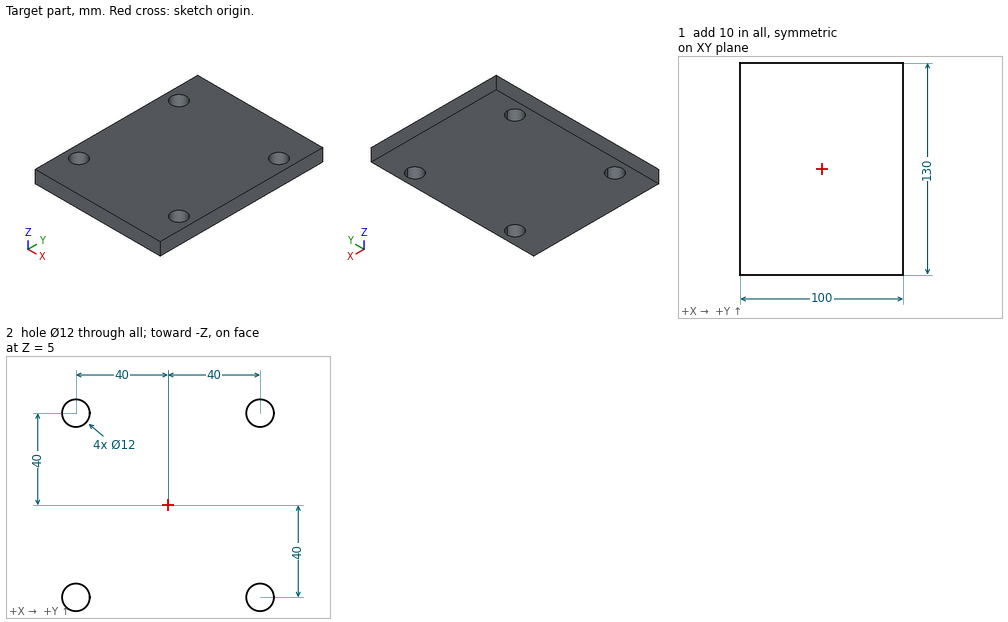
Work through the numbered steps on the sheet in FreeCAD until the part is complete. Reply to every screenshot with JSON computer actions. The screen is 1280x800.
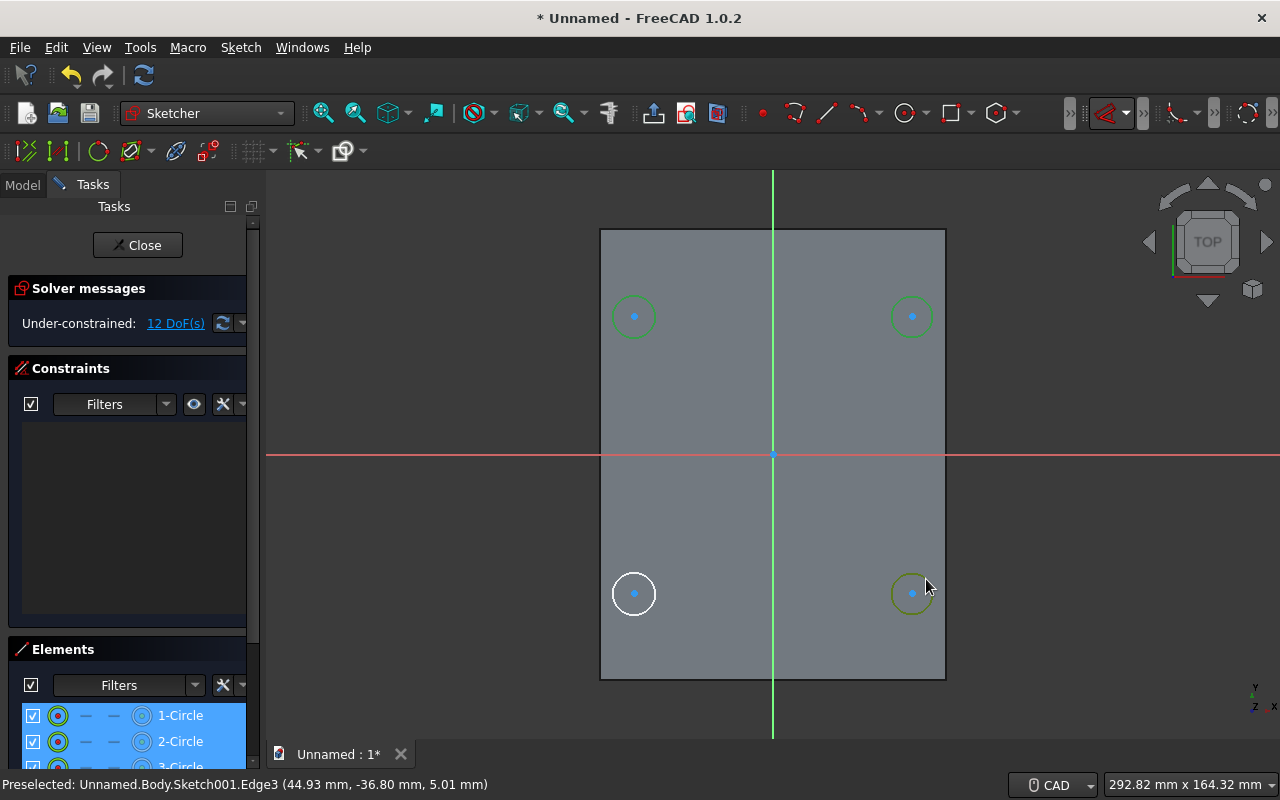
{"action": "left_click", "coordinate": [649, 579]}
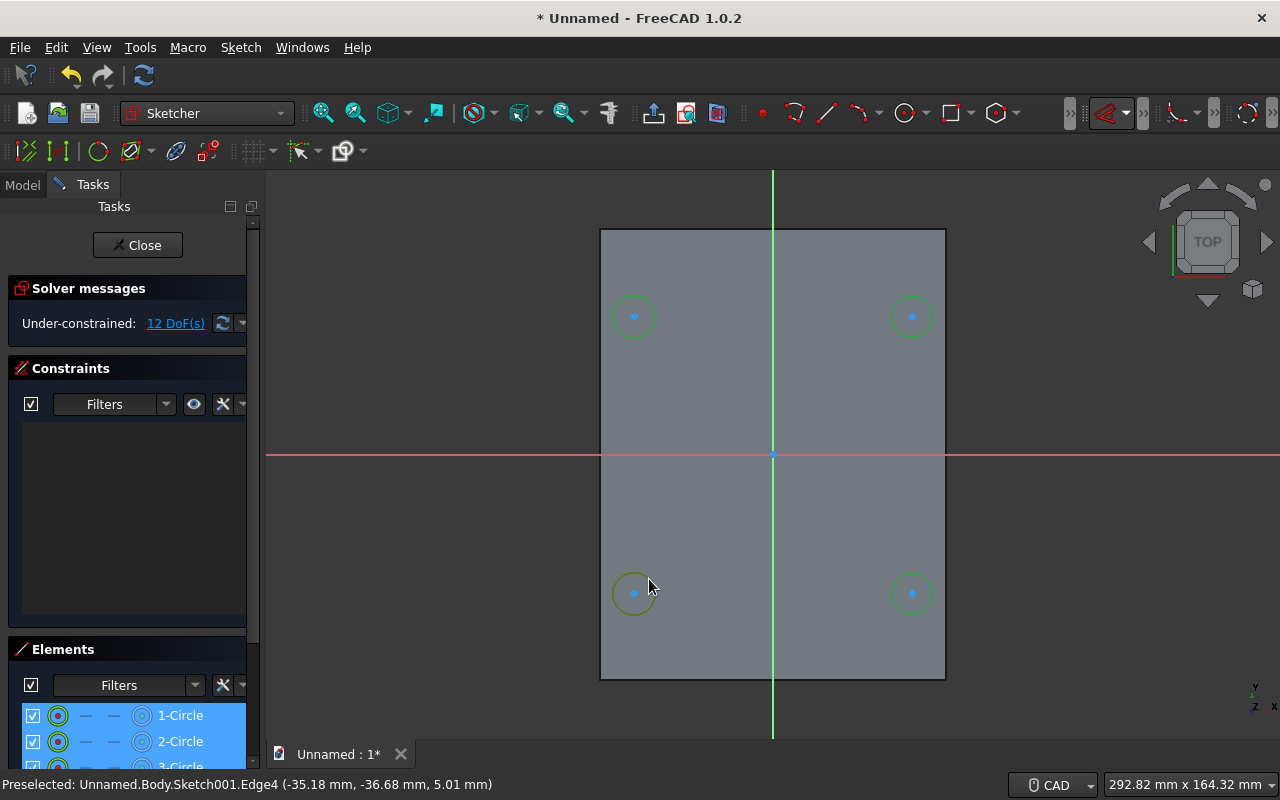
{"action": "key", "text": "e"}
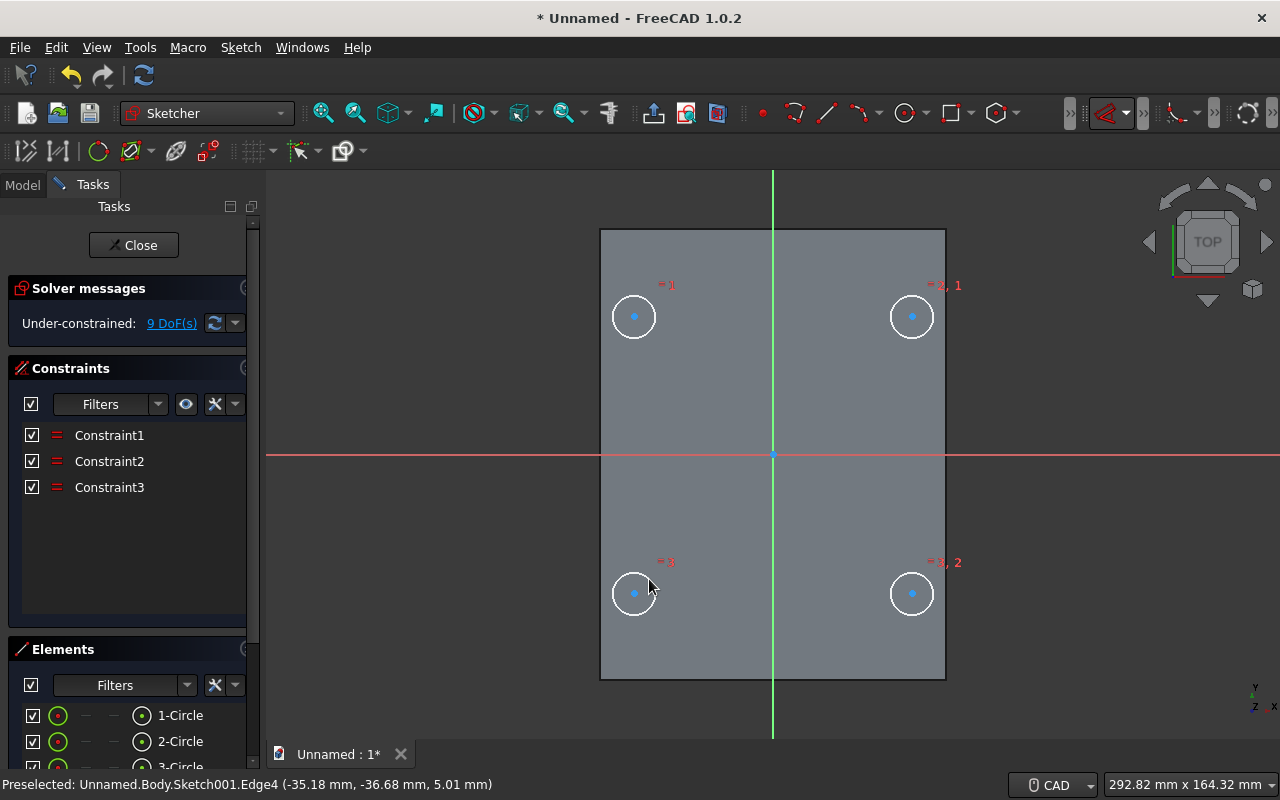
{"action": "left_click", "coordinate": [634, 317]}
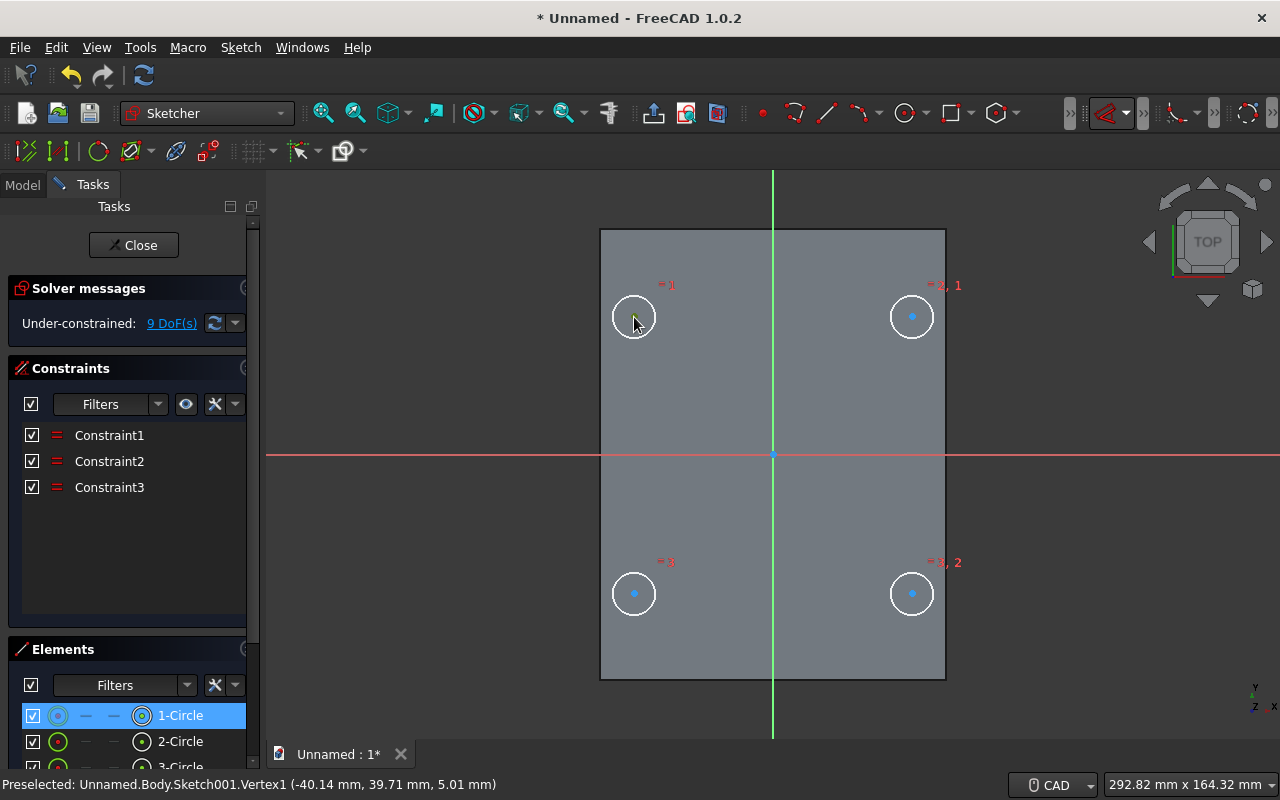
{"action": "left_click", "coordinate": [912, 317]}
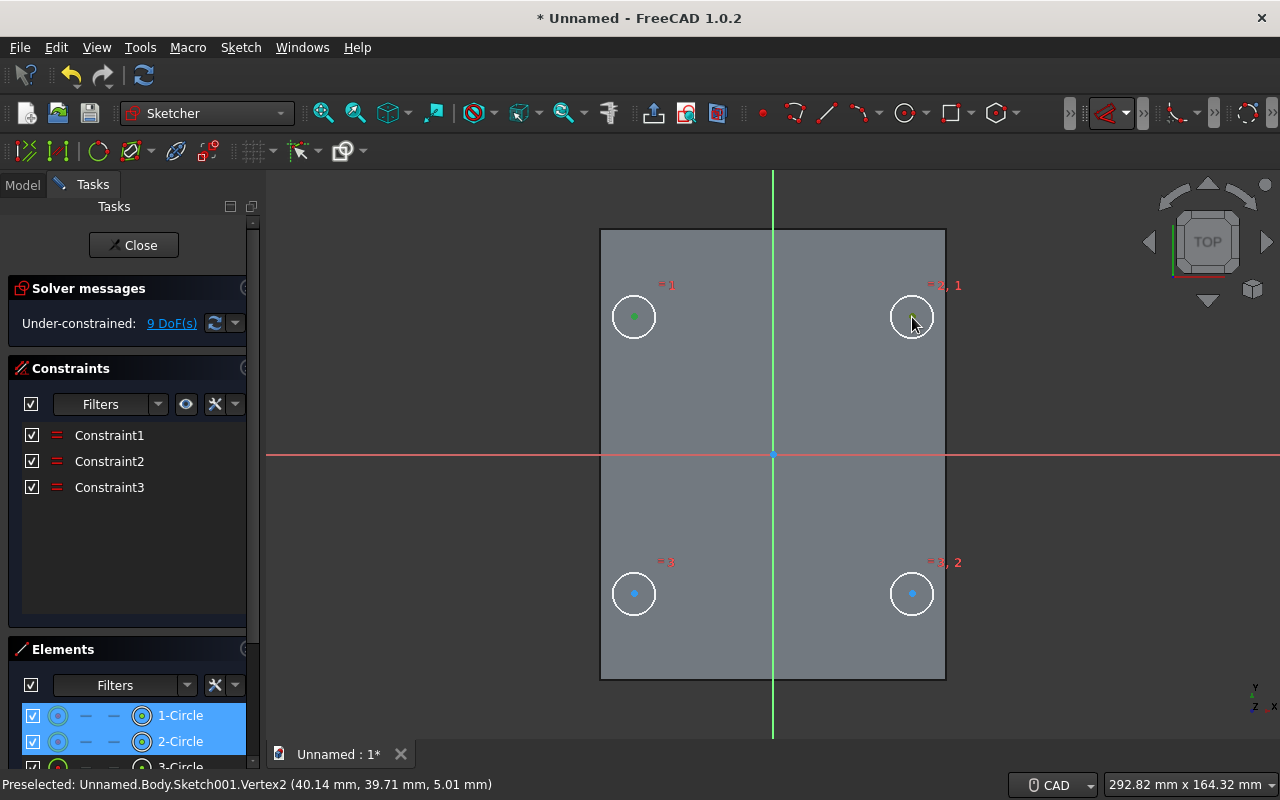
{"action": "key", "text": "h"}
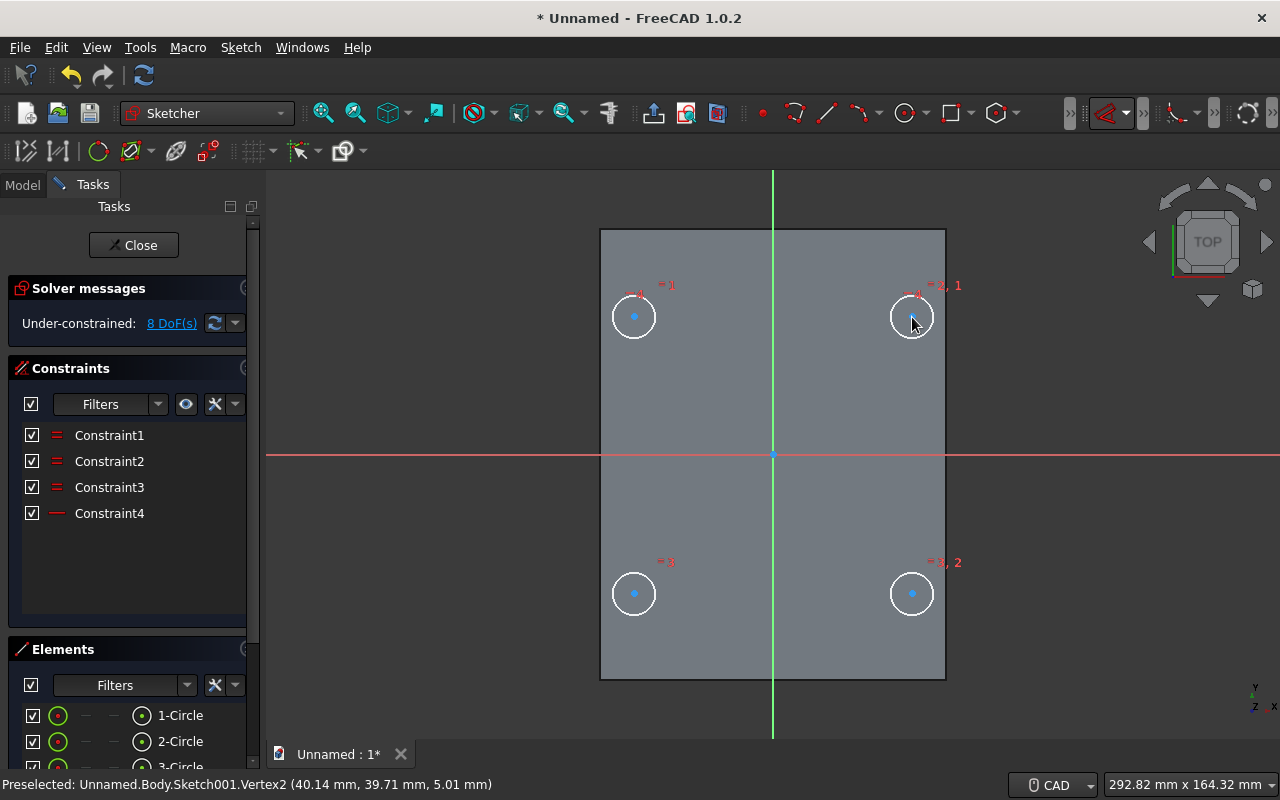
{"action": "left_click", "coordinate": [912, 317]}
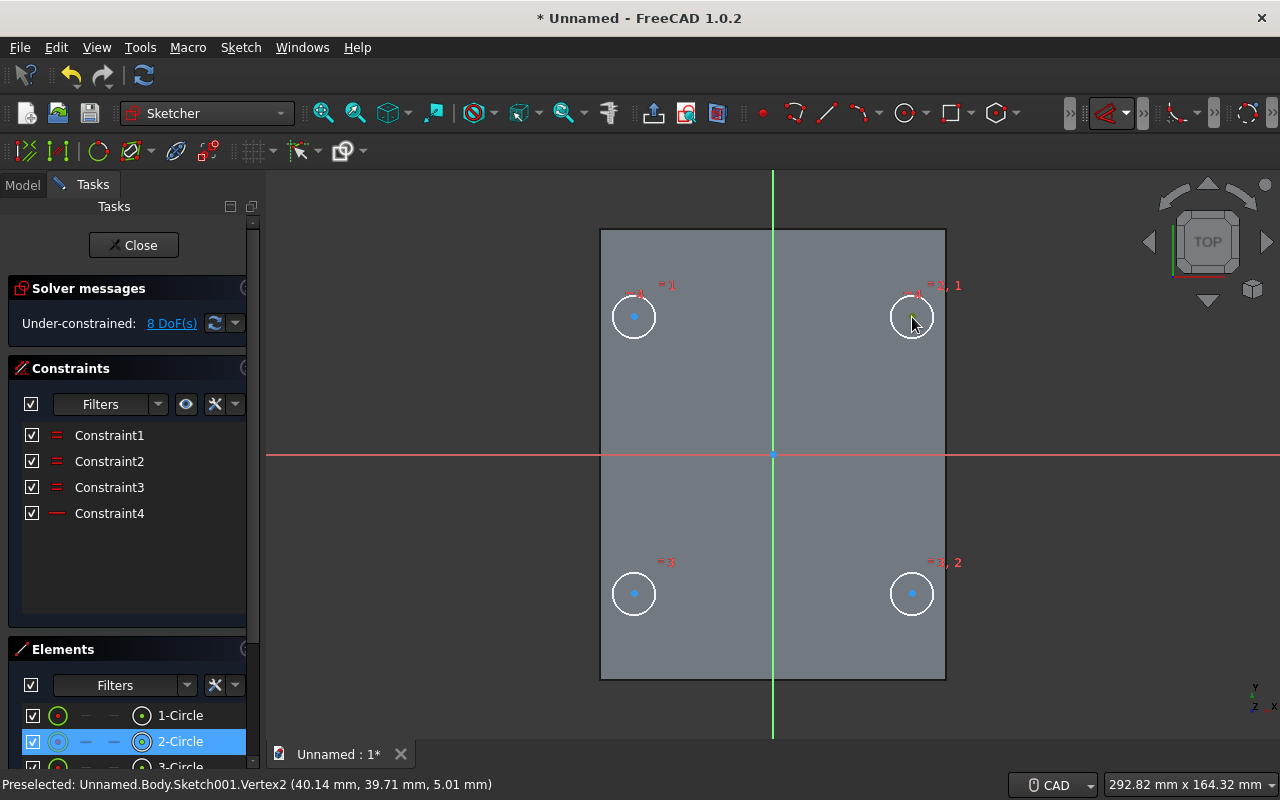
{"action": "left_click", "coordinate": [912, 594]}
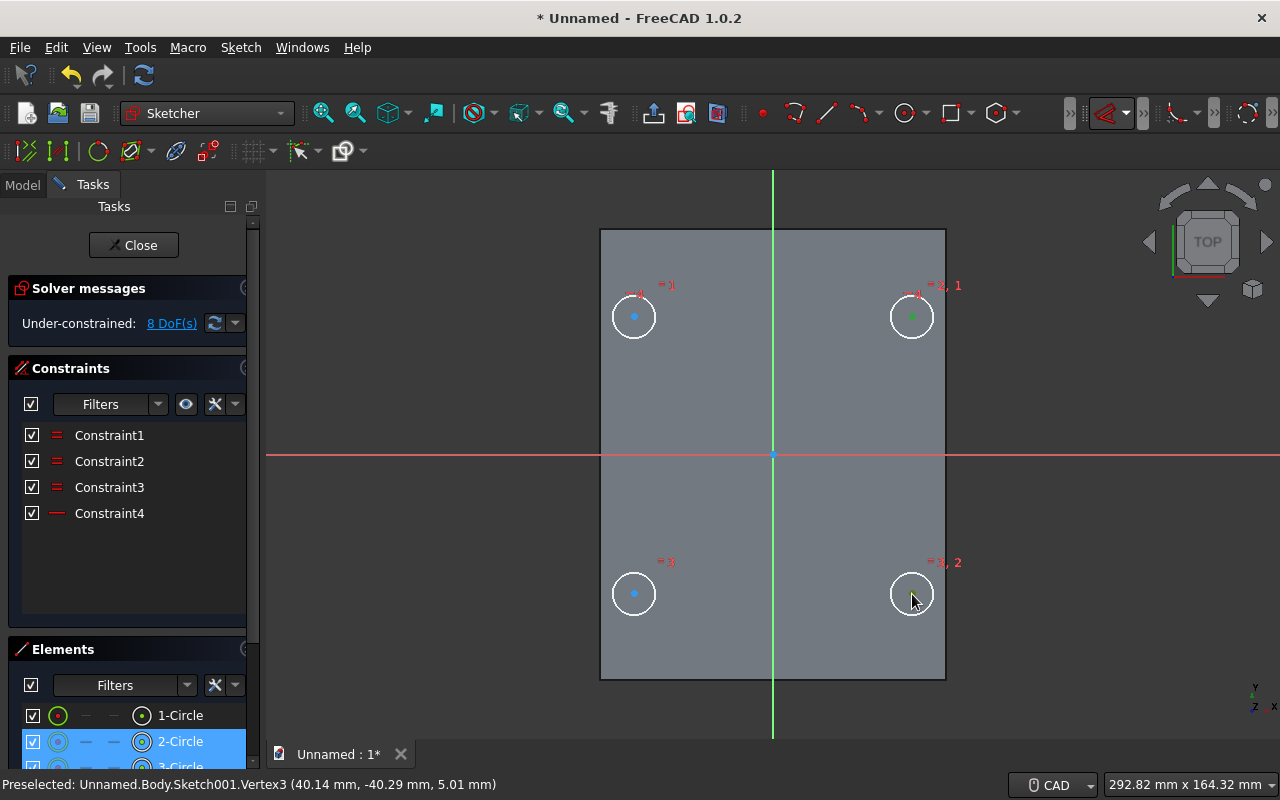
{"action": "key", "text": "v"}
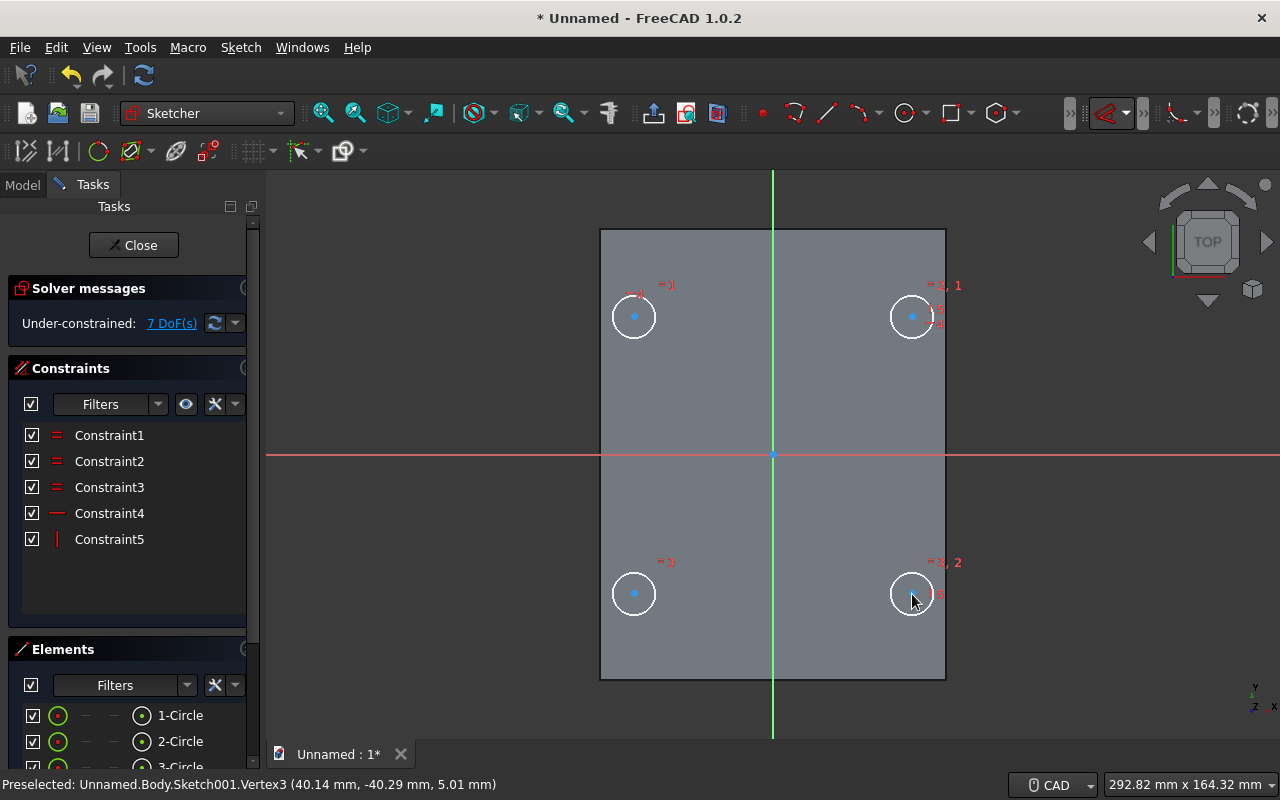
{"action": "left_click", "coordinate": [634, 317]}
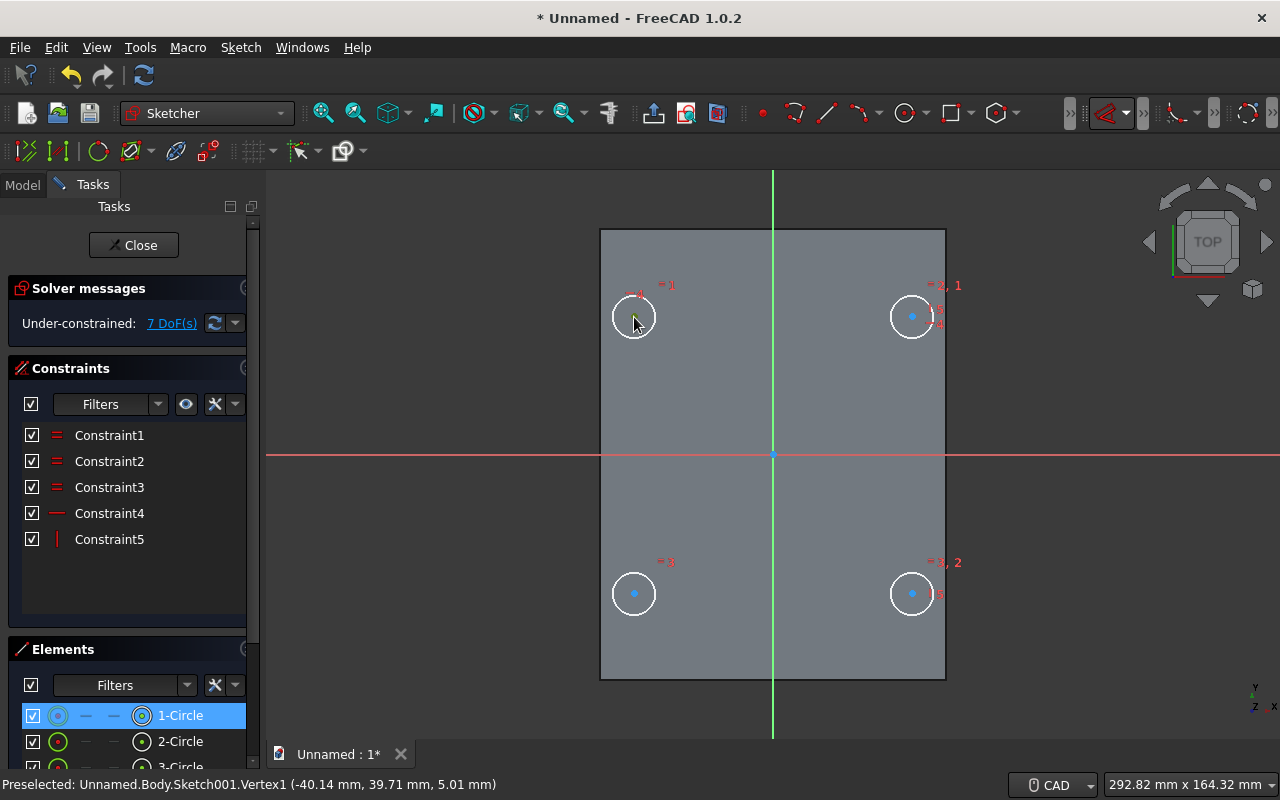
{"action": "left_click", "coordinate": [634, 594]}